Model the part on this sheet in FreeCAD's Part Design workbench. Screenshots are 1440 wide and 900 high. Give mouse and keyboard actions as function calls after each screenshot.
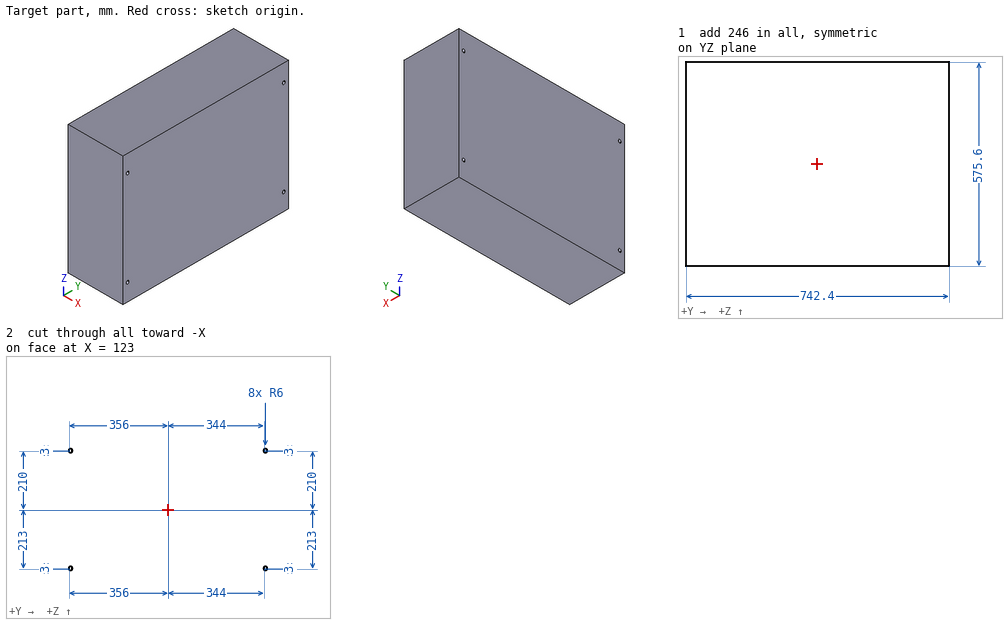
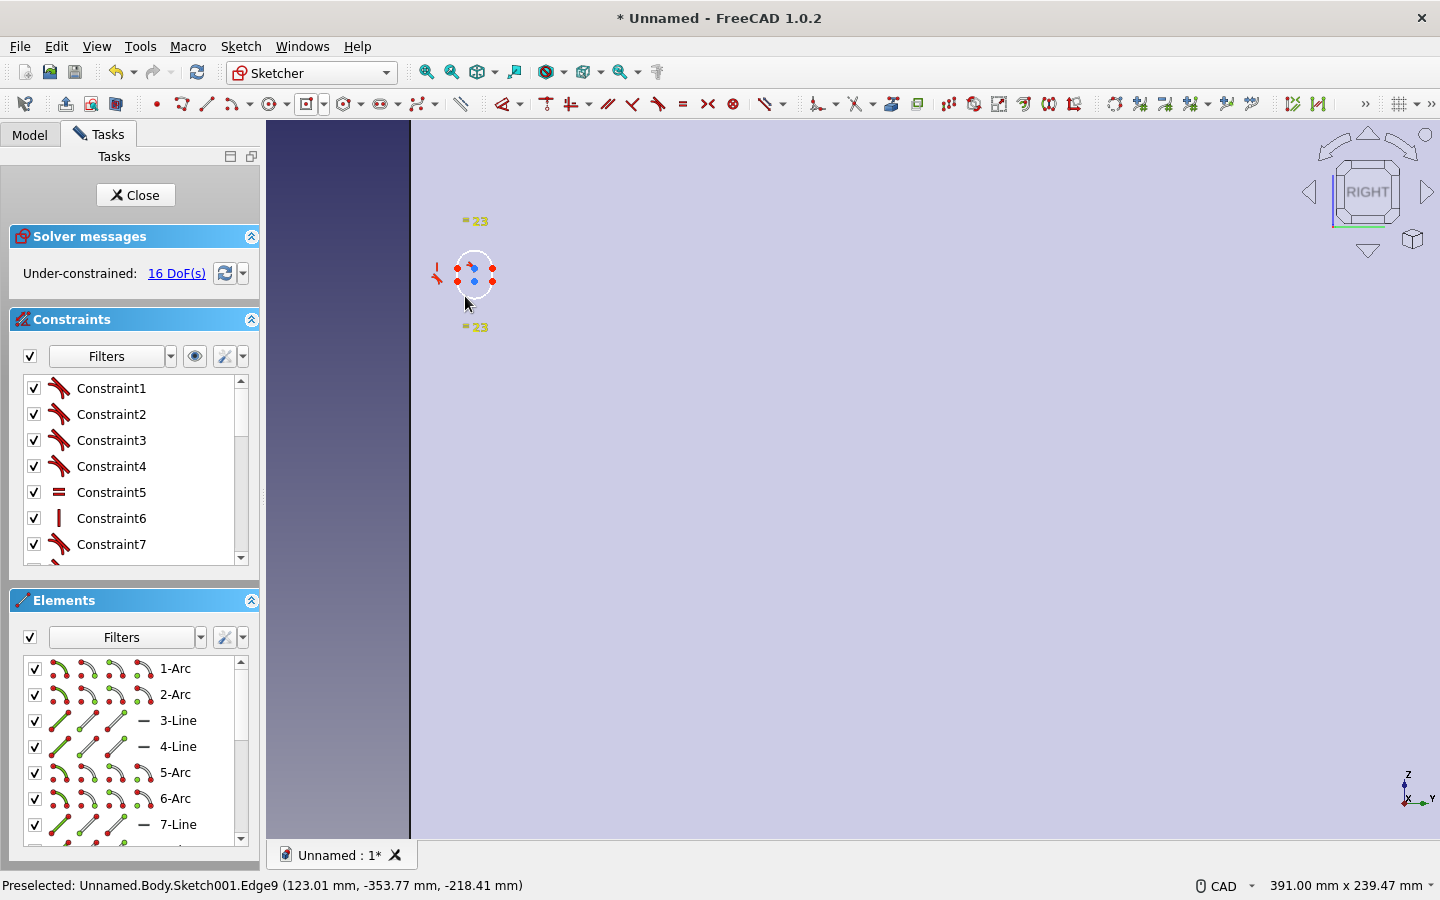
click(464, 295)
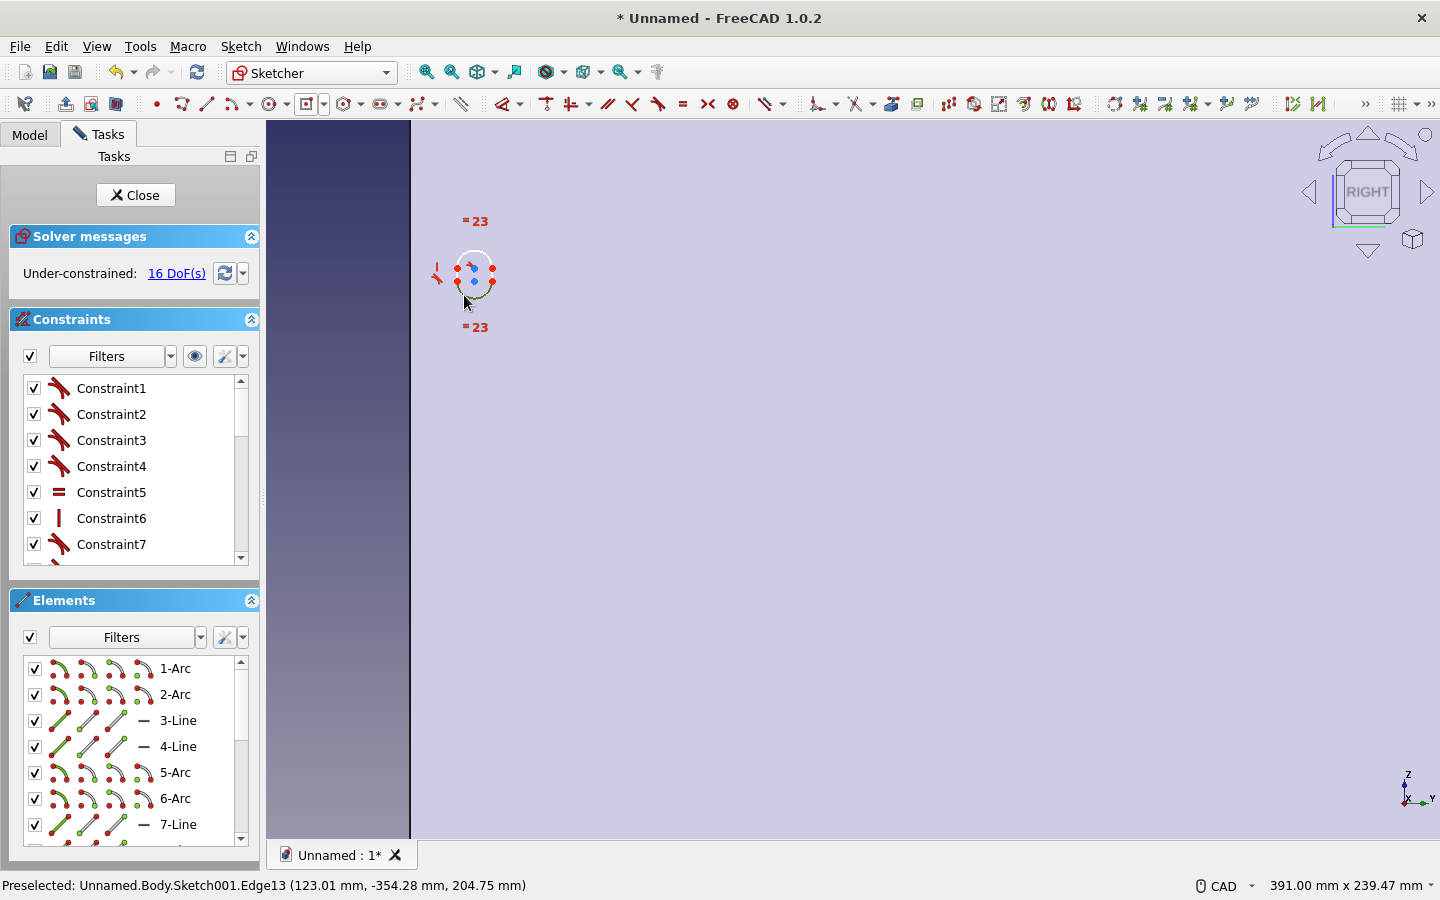
click(683, 104)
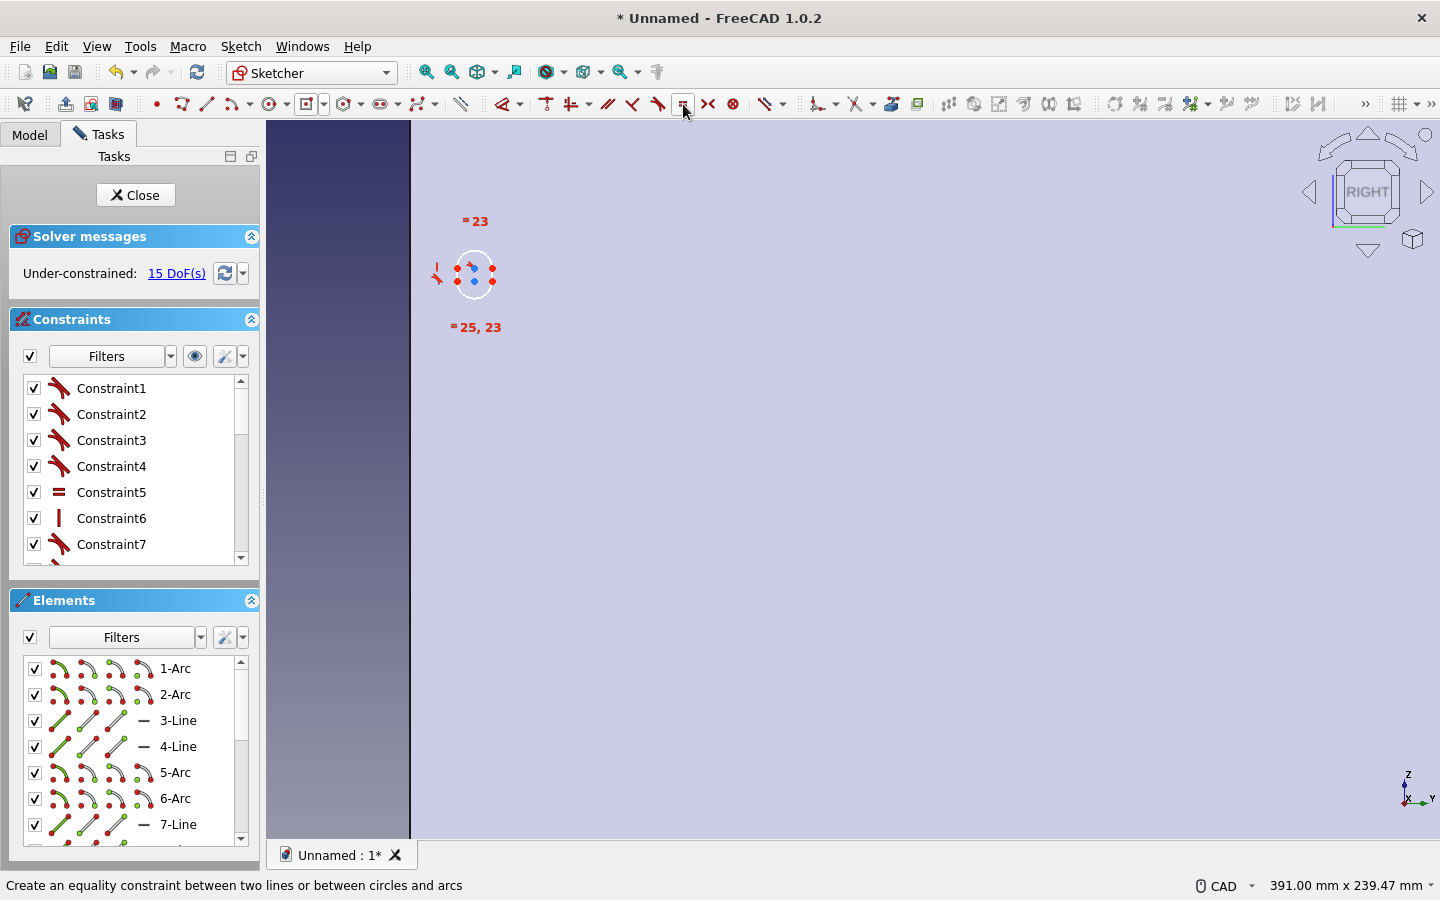
scroll(465, 295, down, 6)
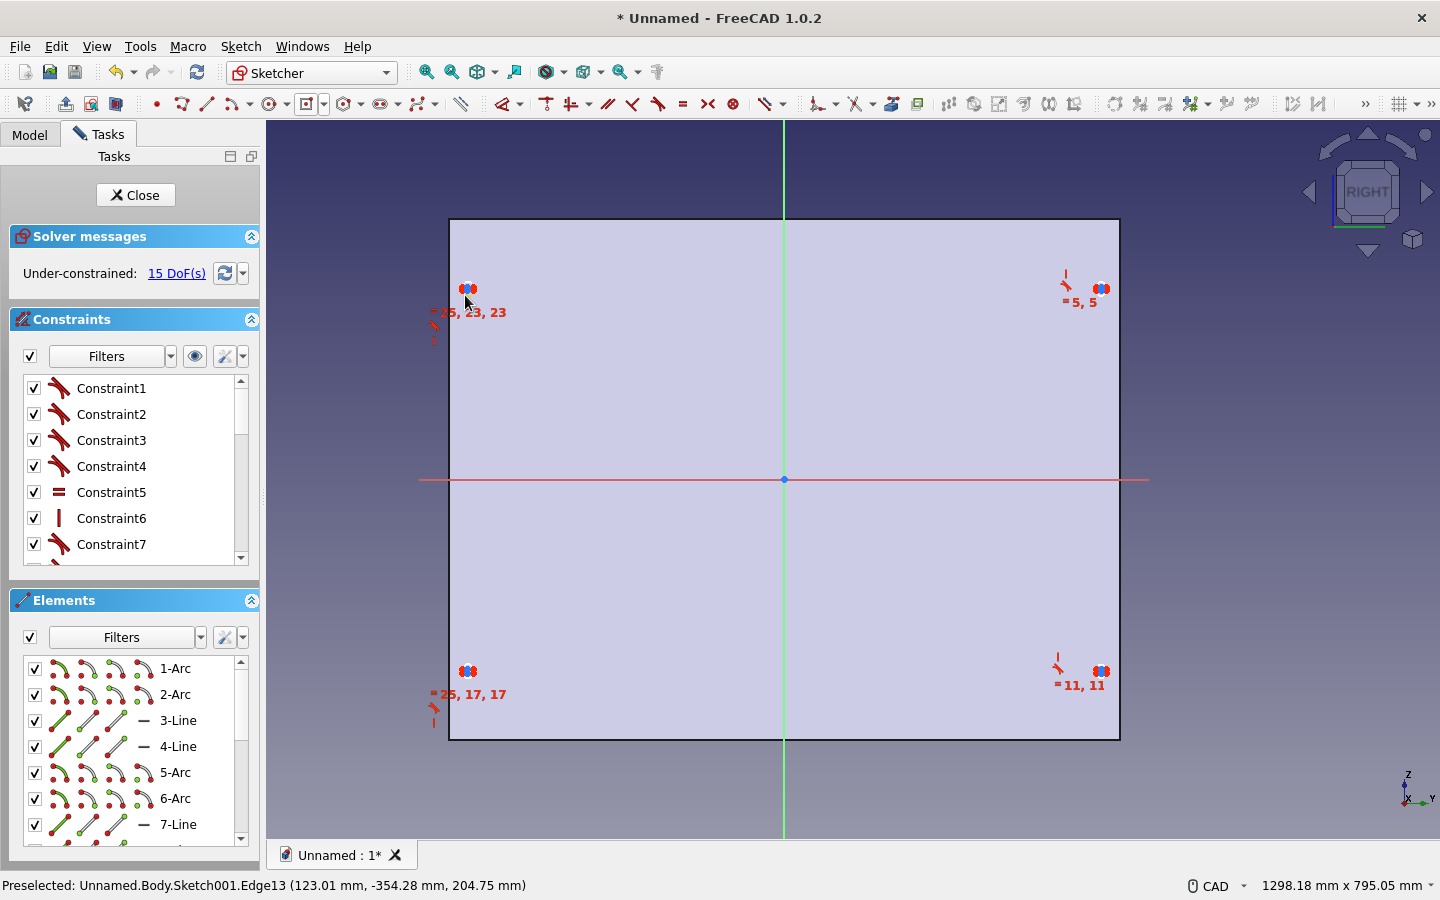
scroll(1098, 295, up, 6)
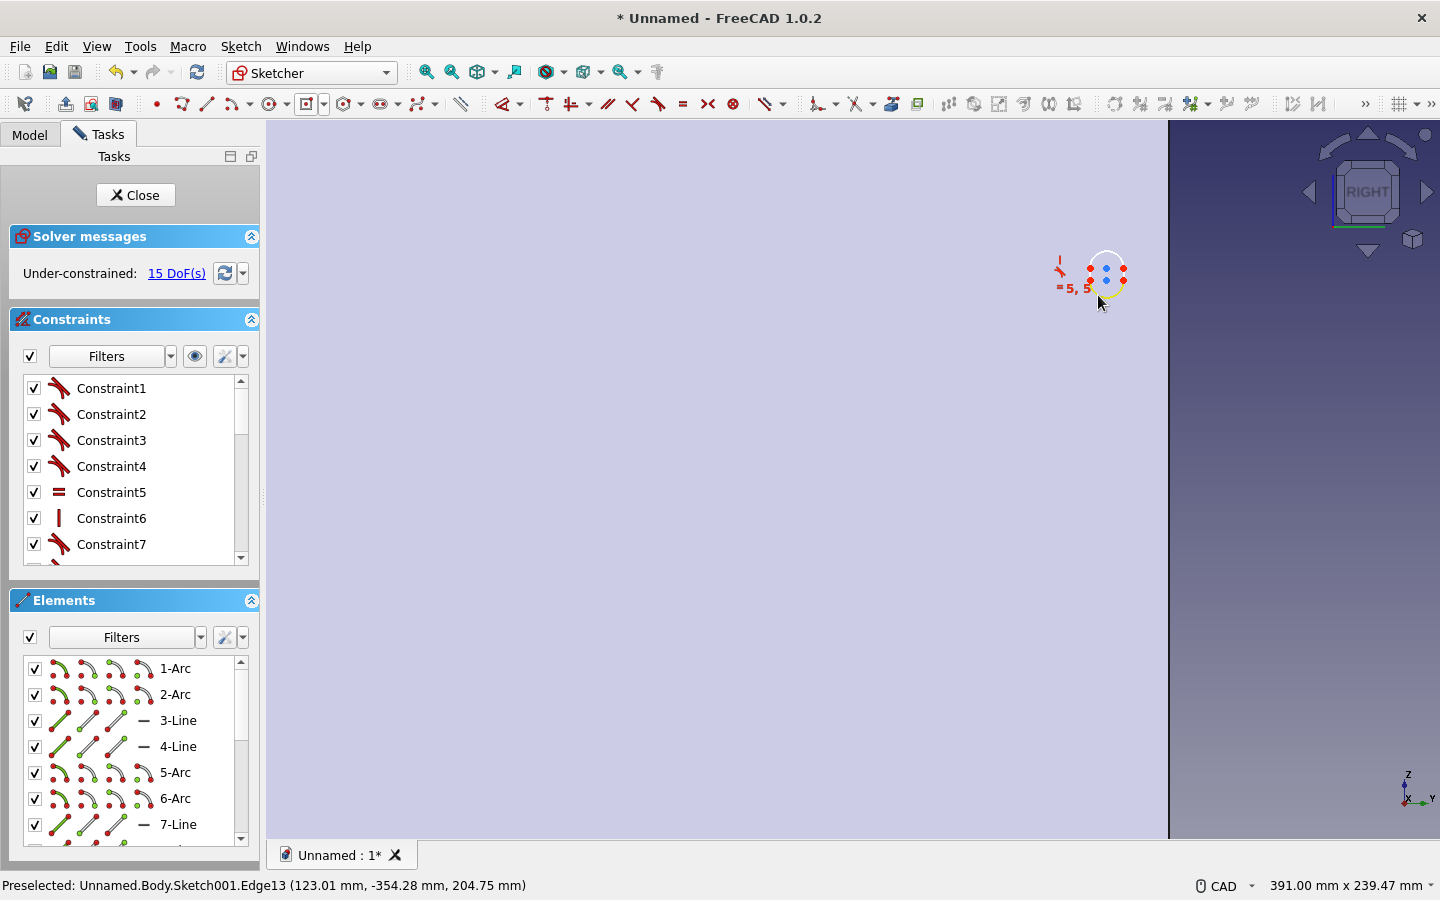
click(1097, 295)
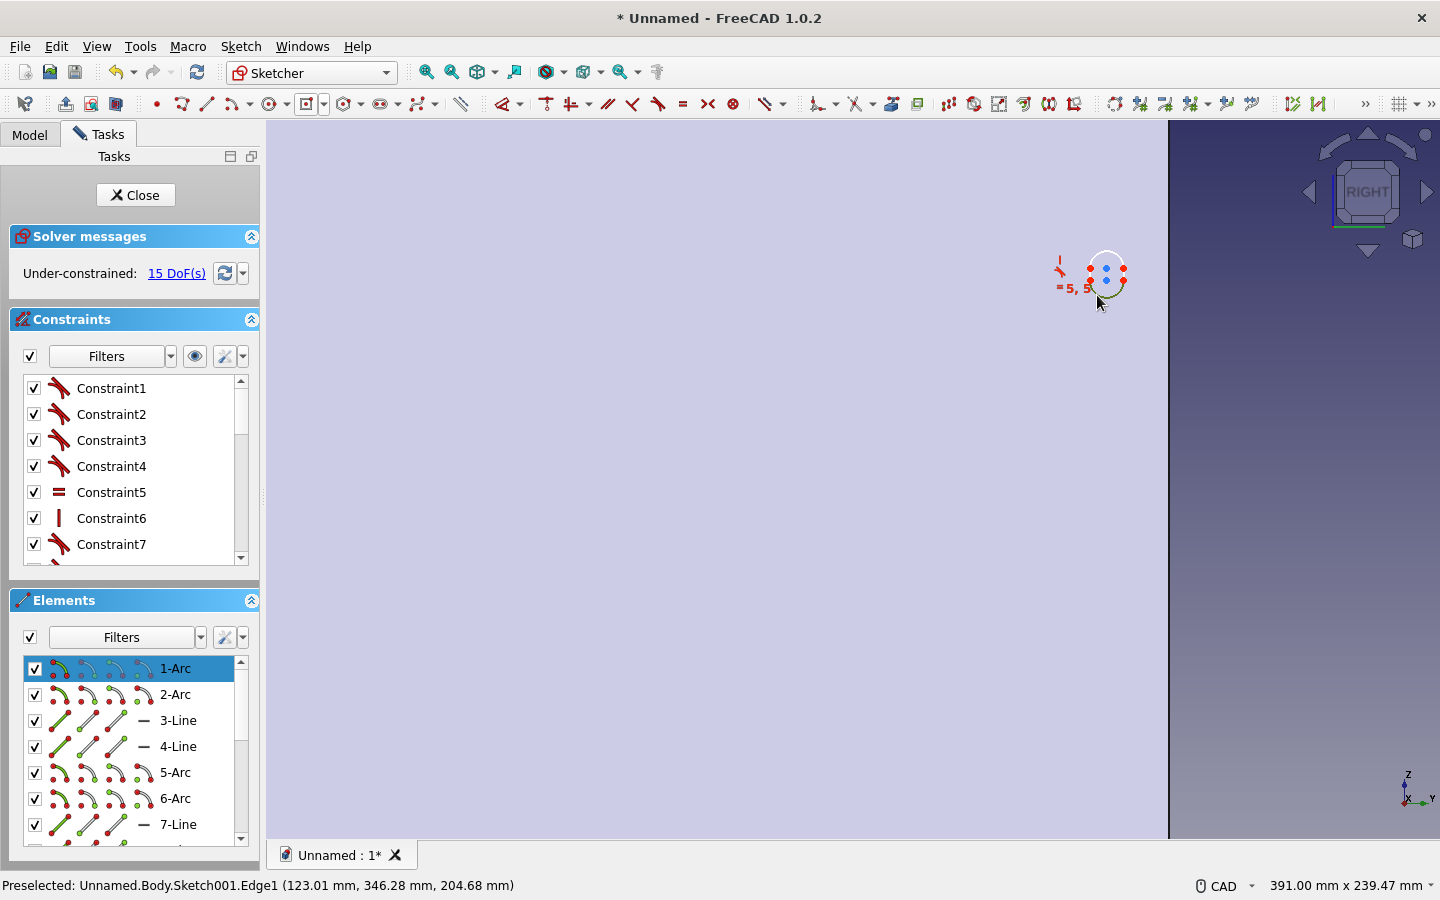
scroll(1099, 295, down, 6)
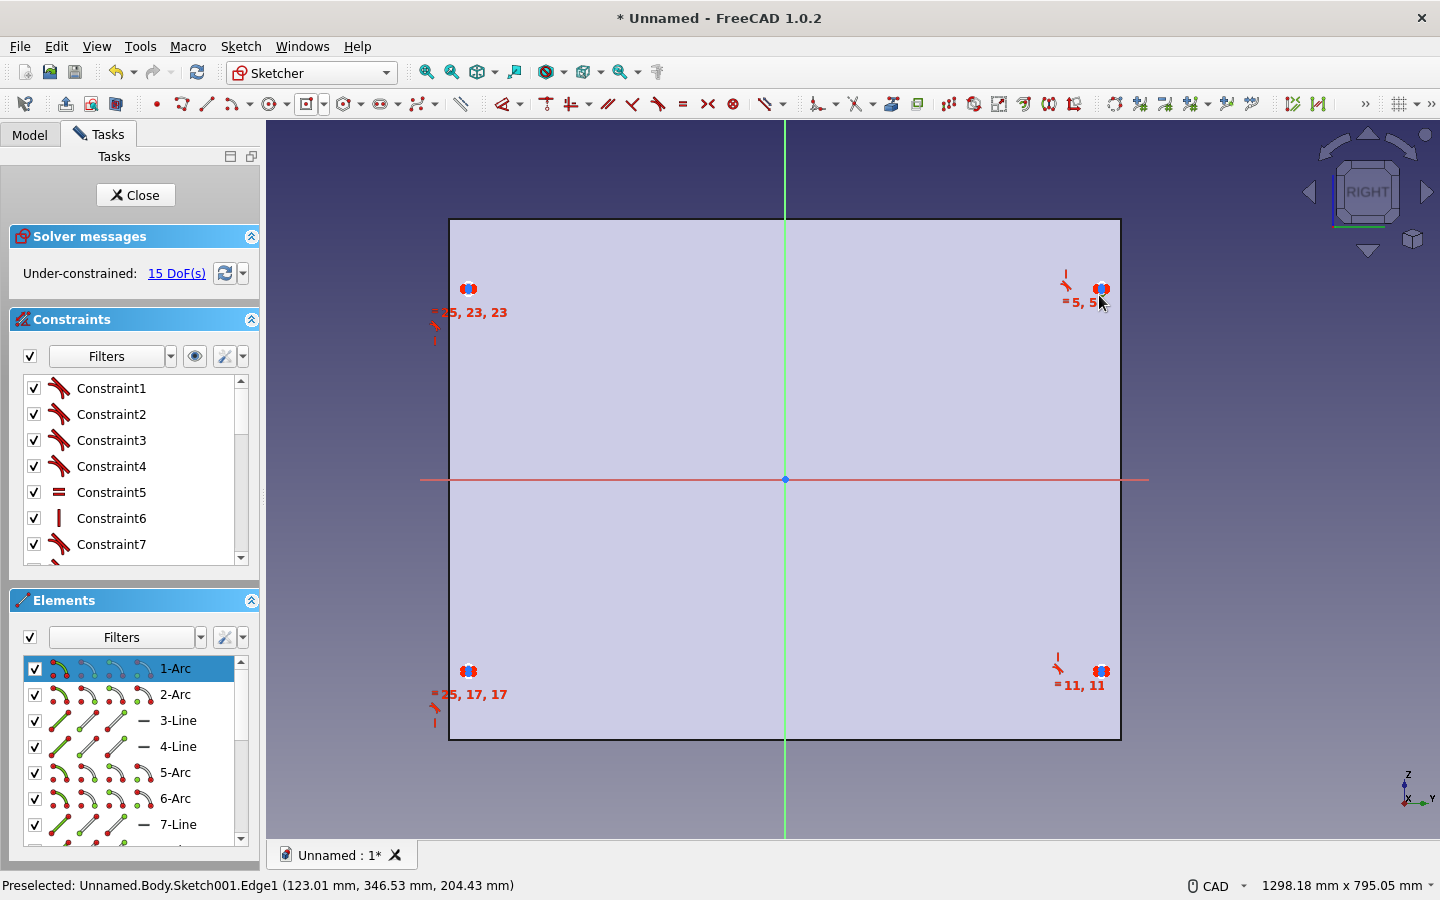
scroll(1105, 665, up, 6)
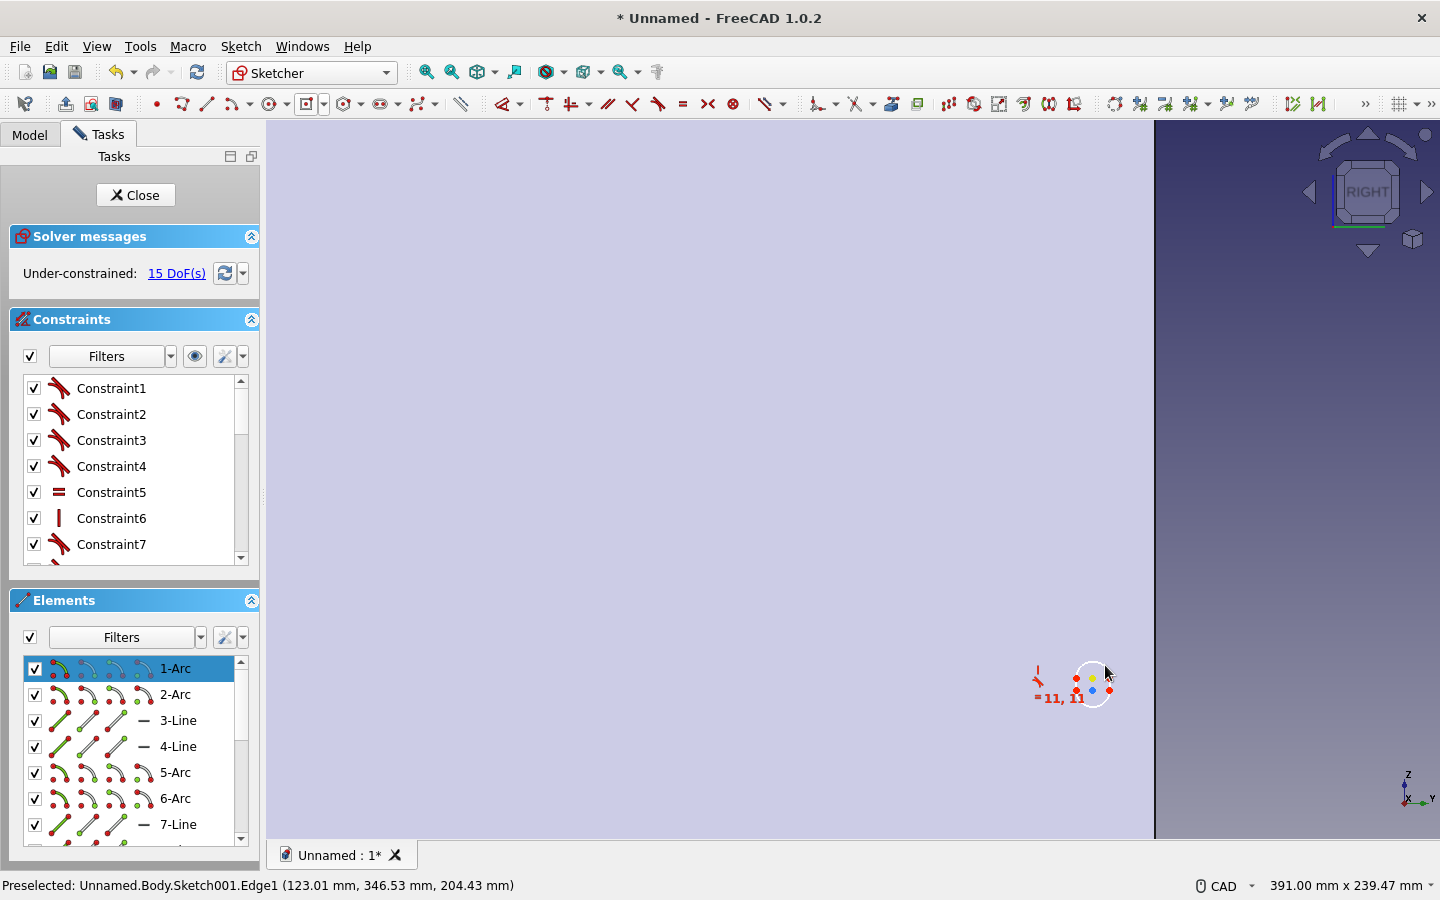
click(1103, 665)